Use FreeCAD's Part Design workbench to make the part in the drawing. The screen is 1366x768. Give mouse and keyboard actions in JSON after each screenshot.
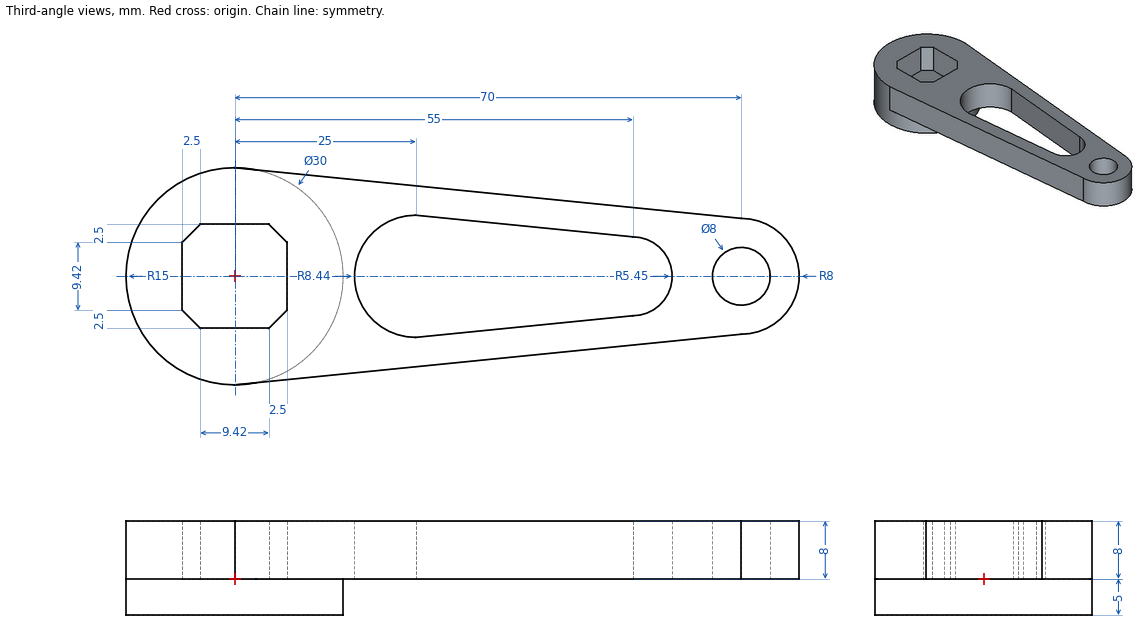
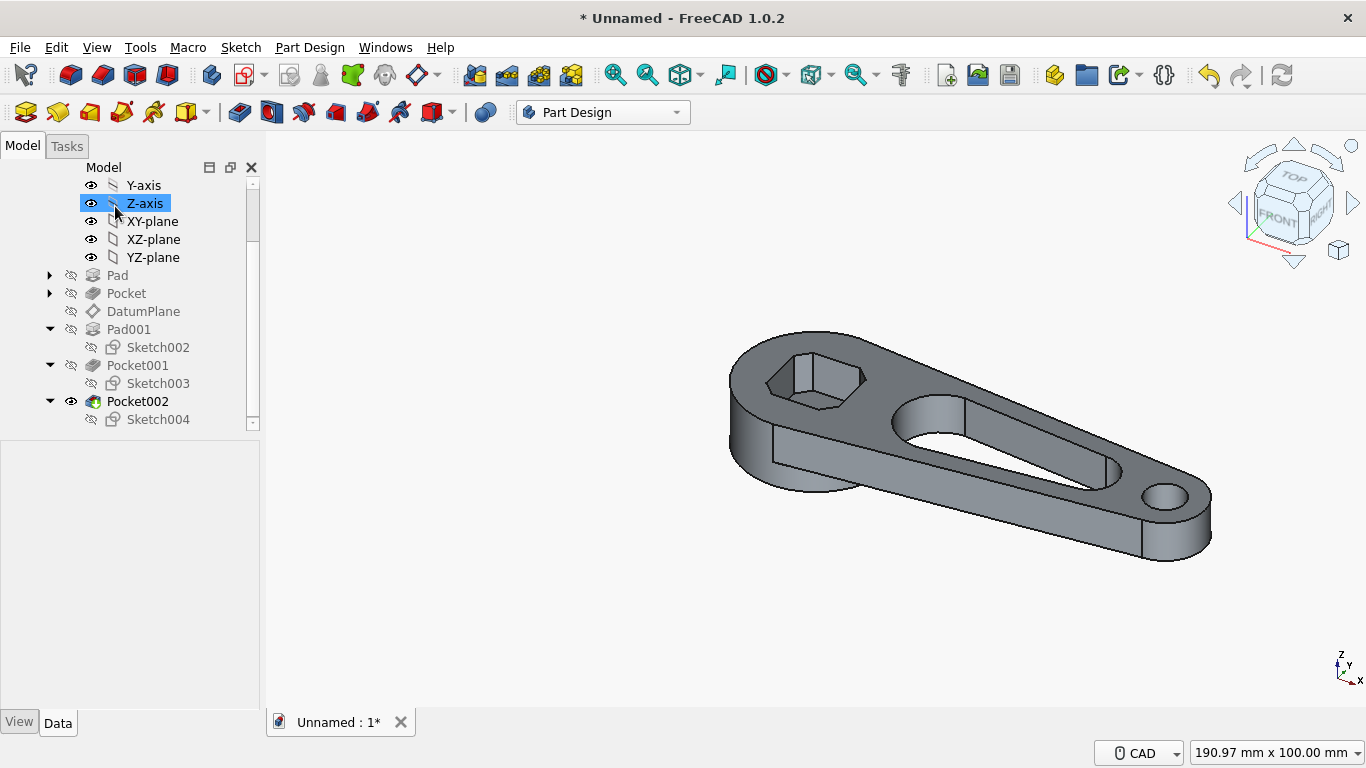
{"action": "key", "text": "0"}